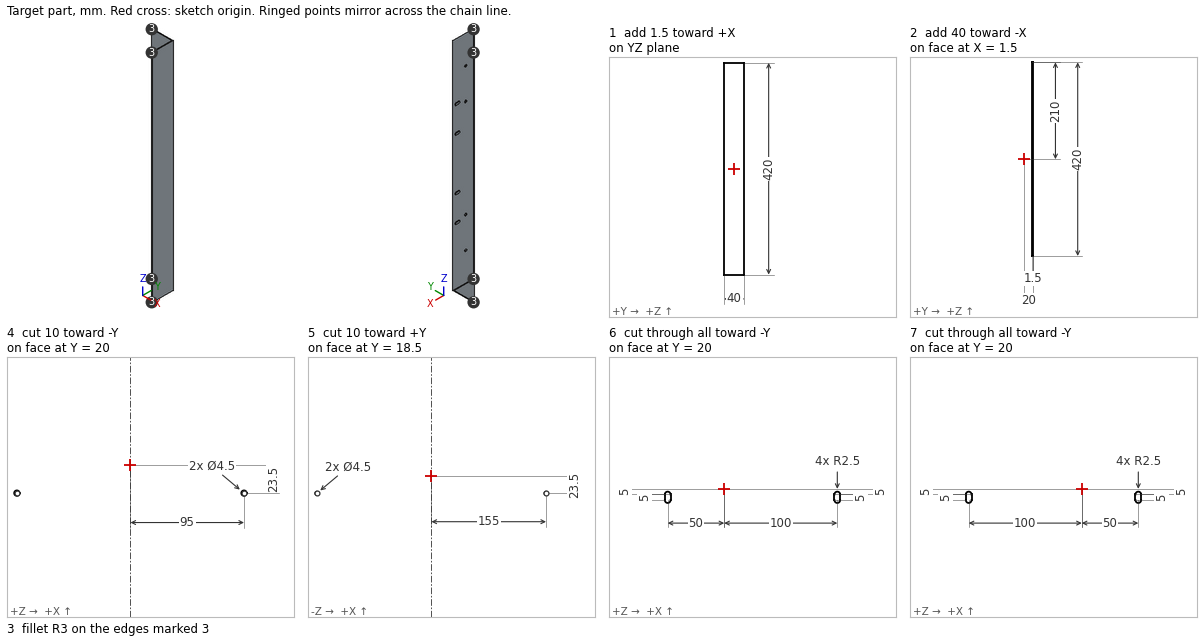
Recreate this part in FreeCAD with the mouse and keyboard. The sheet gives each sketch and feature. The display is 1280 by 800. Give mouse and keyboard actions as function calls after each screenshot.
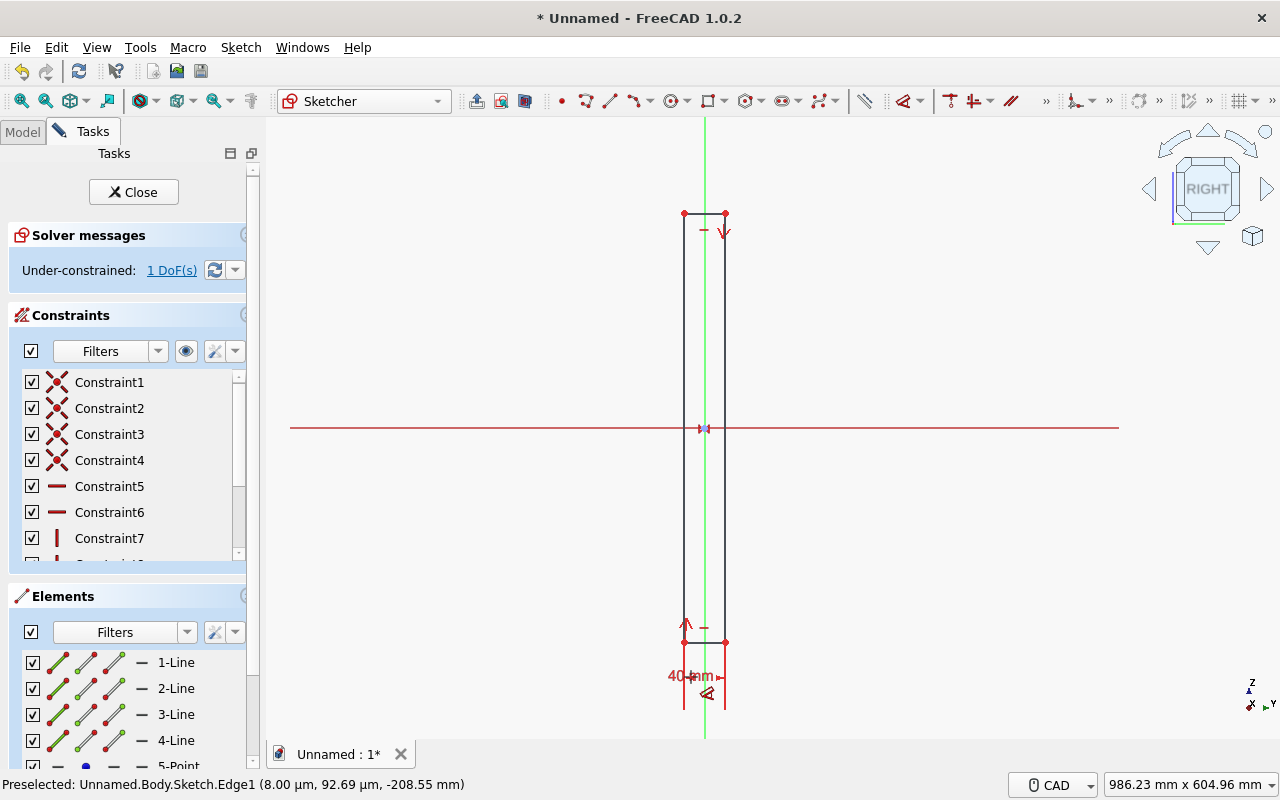
click(725, 514)
click(759, 330)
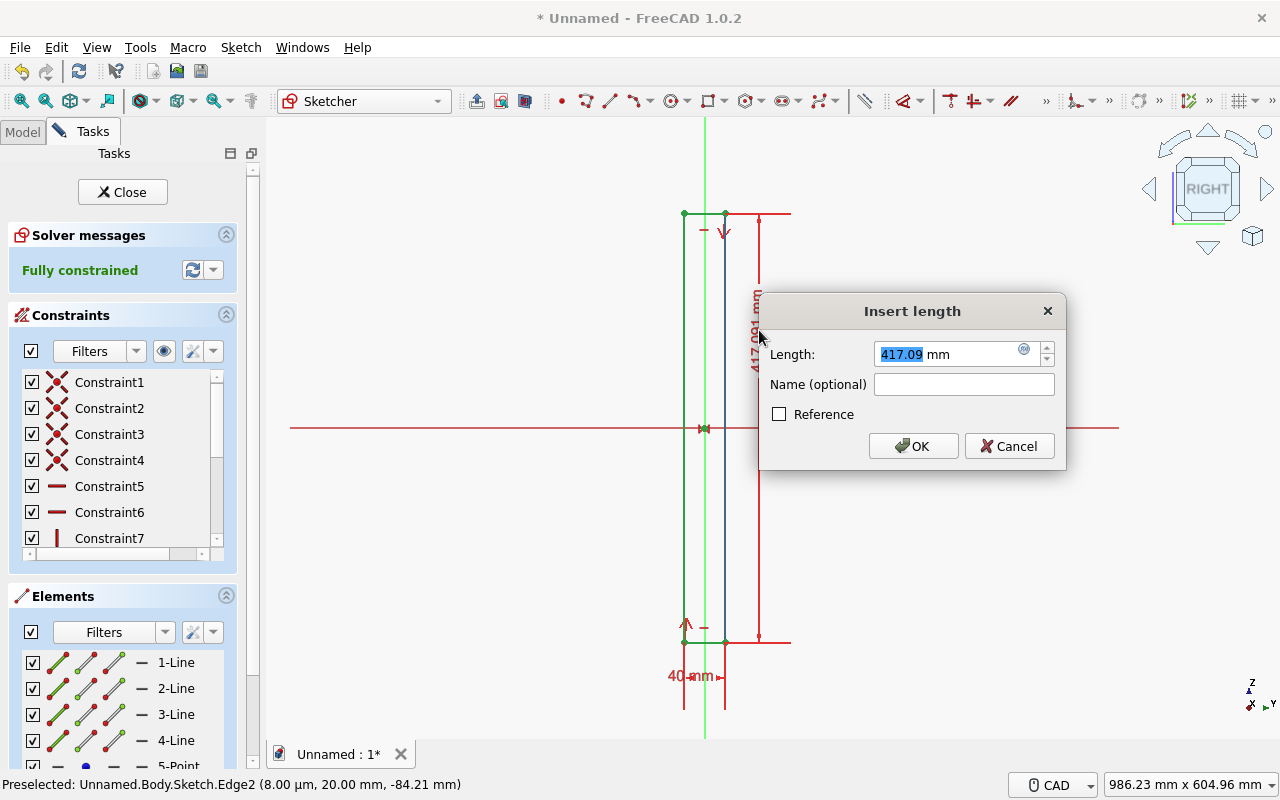
text(420)
key(Return)
key(Escape)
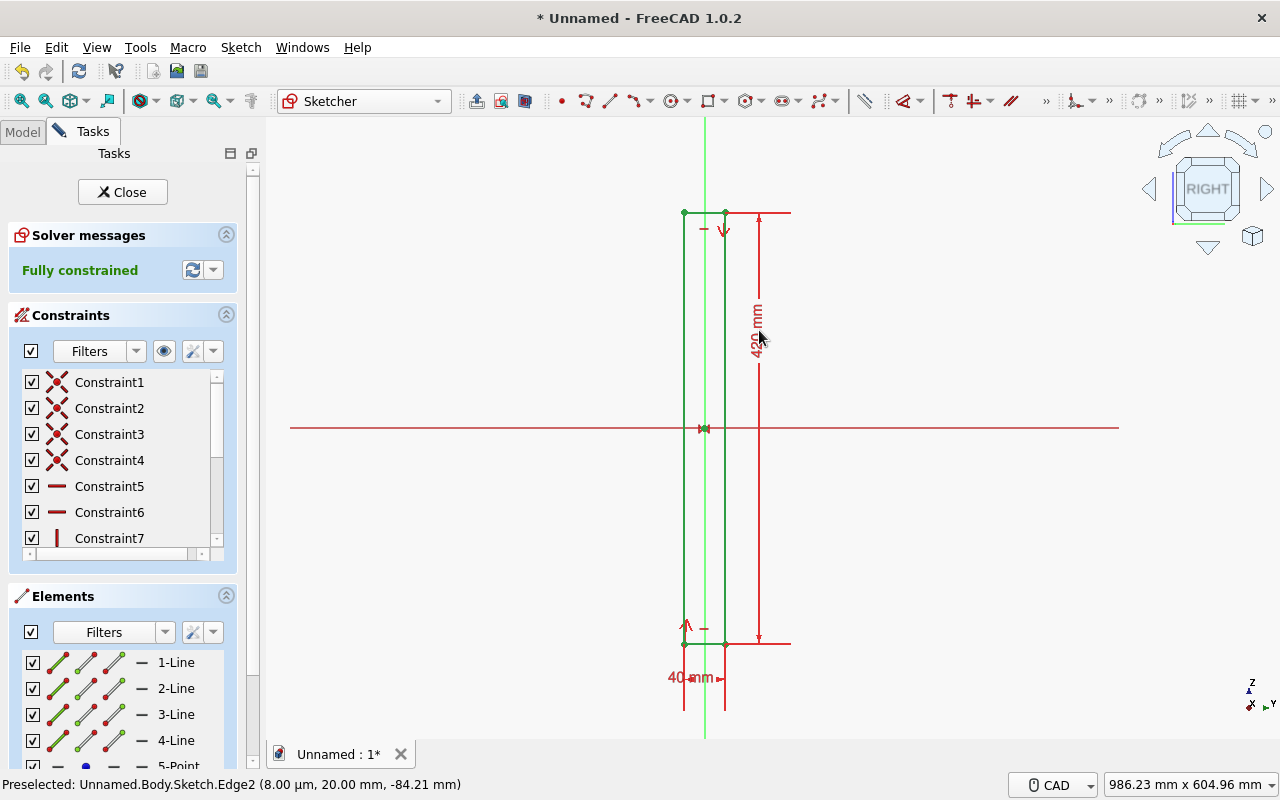
click(123, 192)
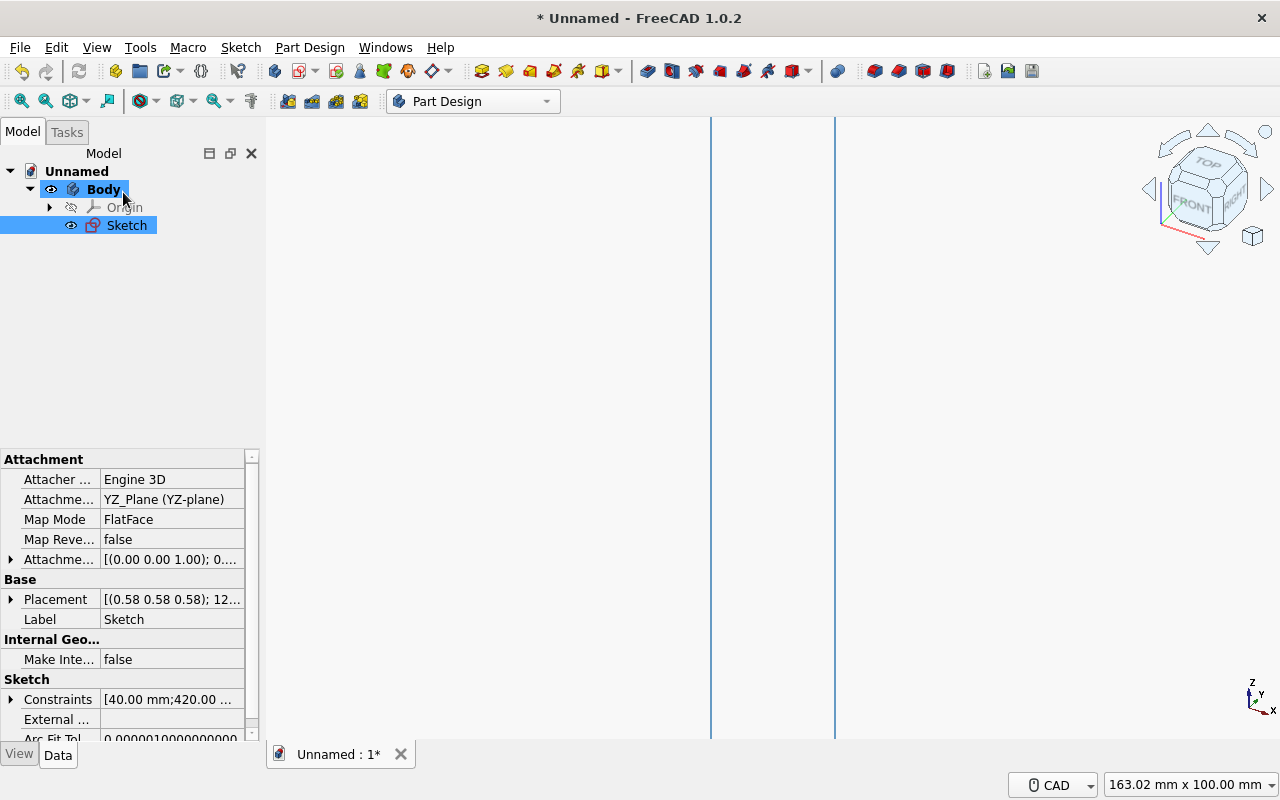
click(482, 72)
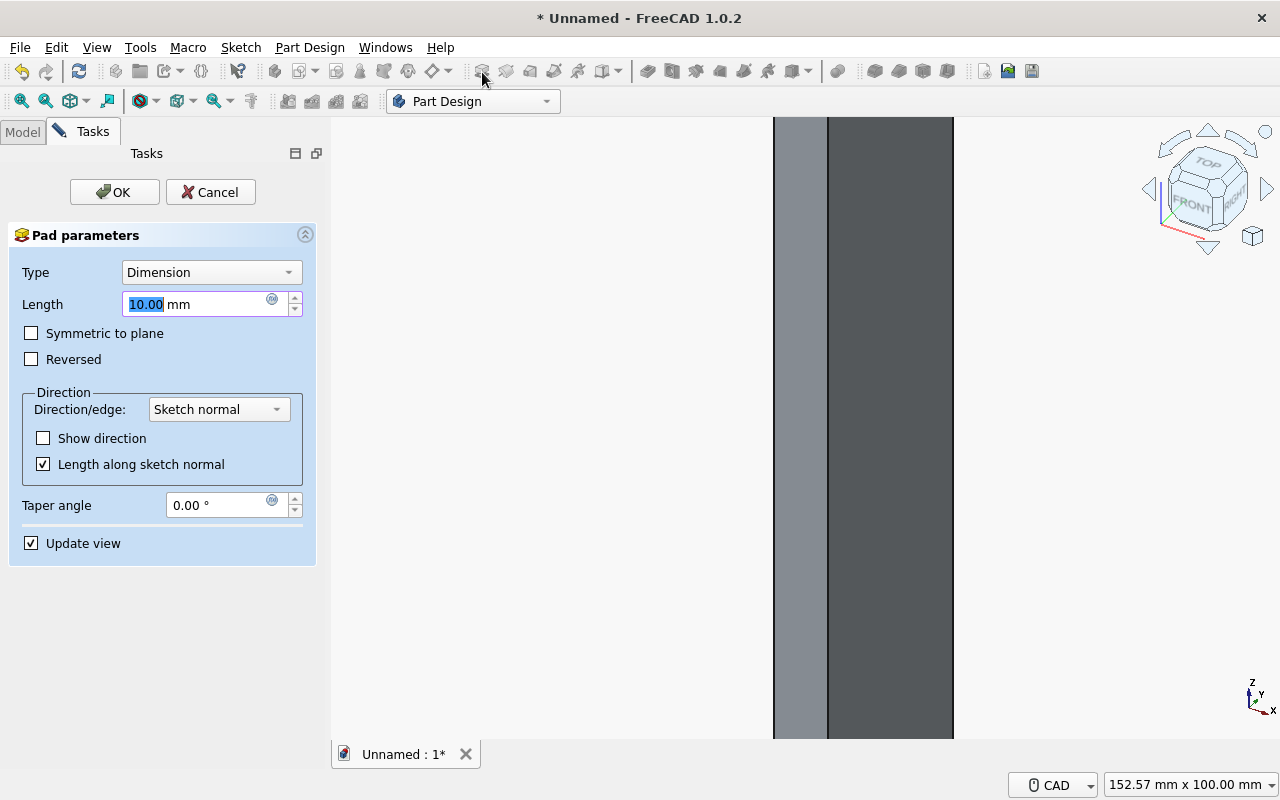
text(1.5)
key(Tab)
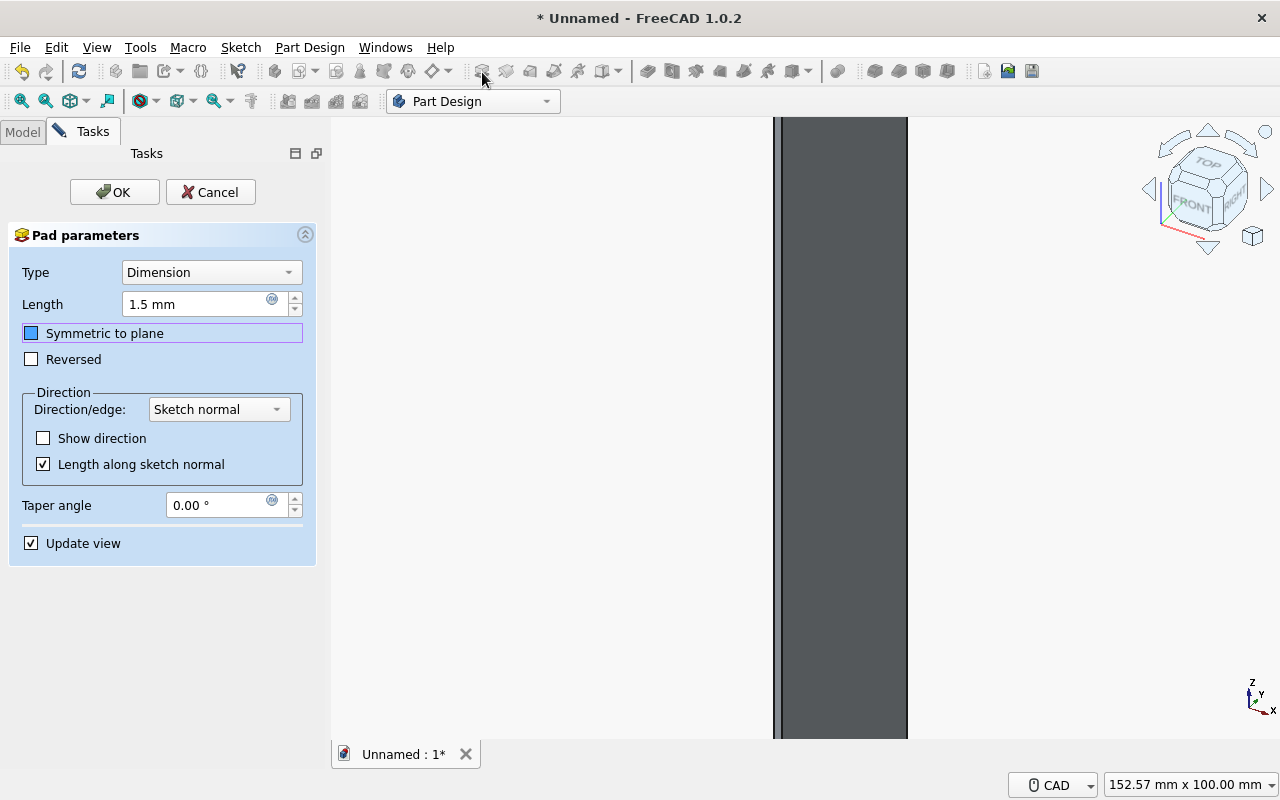
click(115, 192)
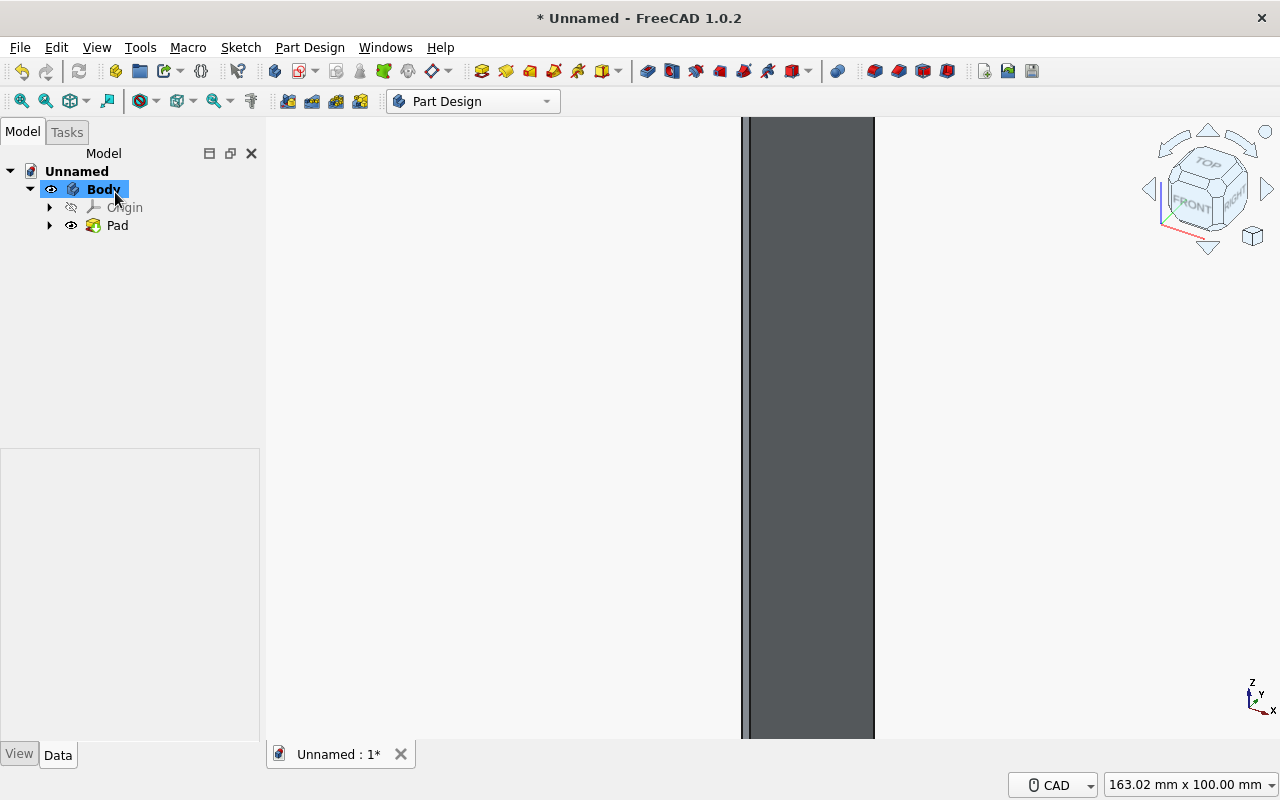
click(22, 102)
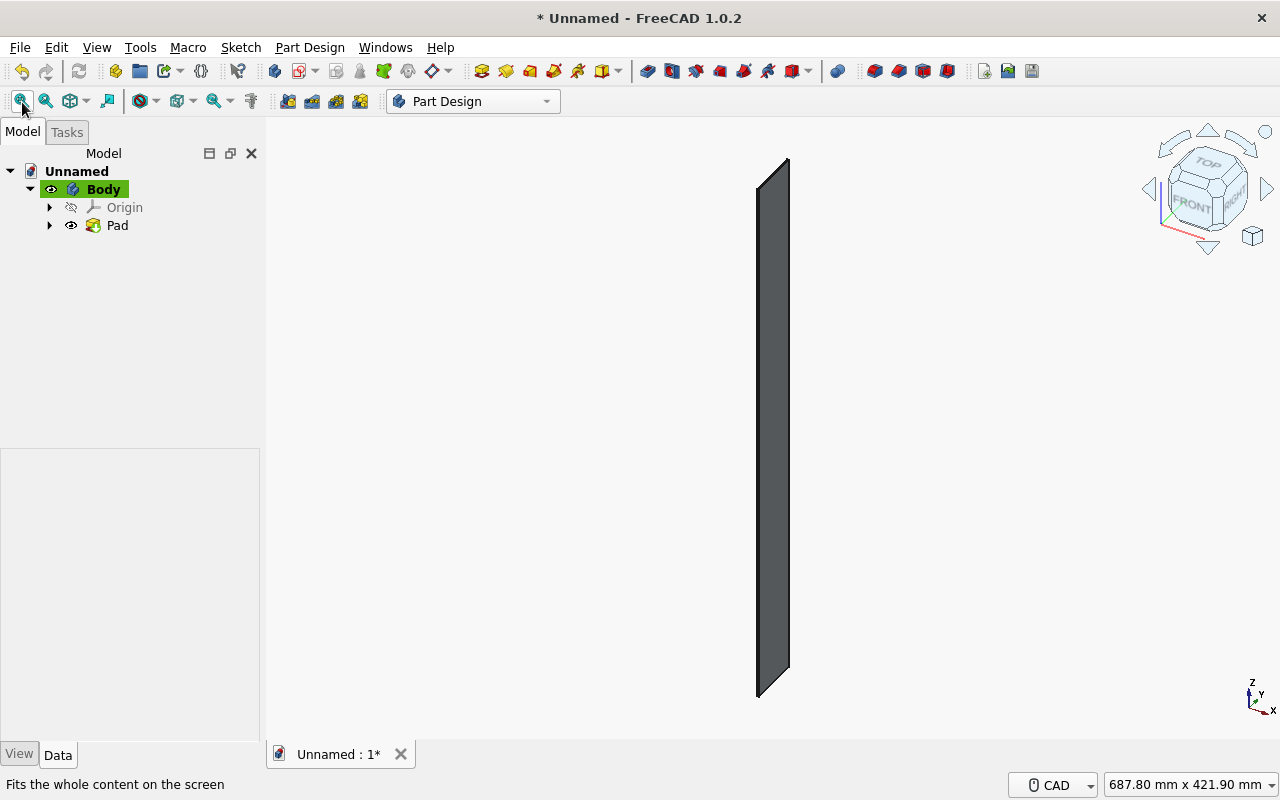
click(774, 427)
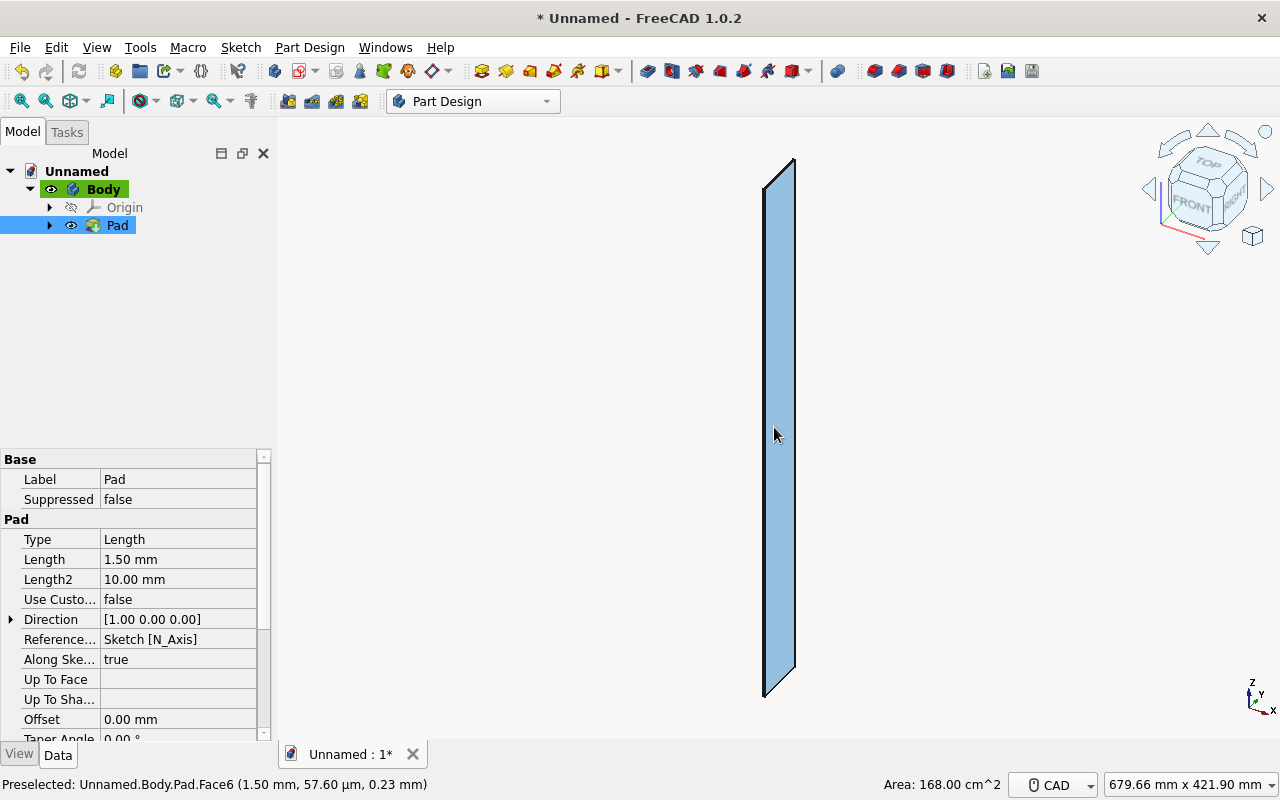
click(300, 72)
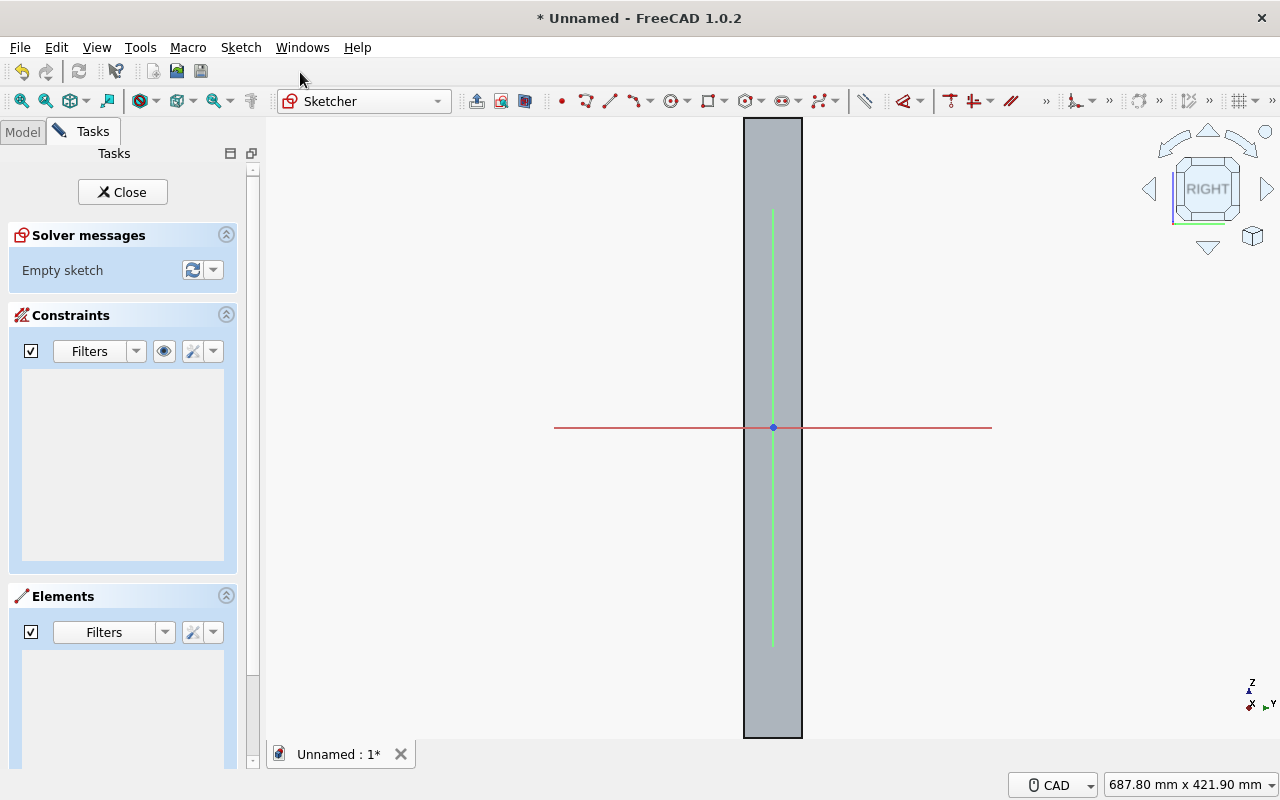
scroll(535, 428, down, 2)